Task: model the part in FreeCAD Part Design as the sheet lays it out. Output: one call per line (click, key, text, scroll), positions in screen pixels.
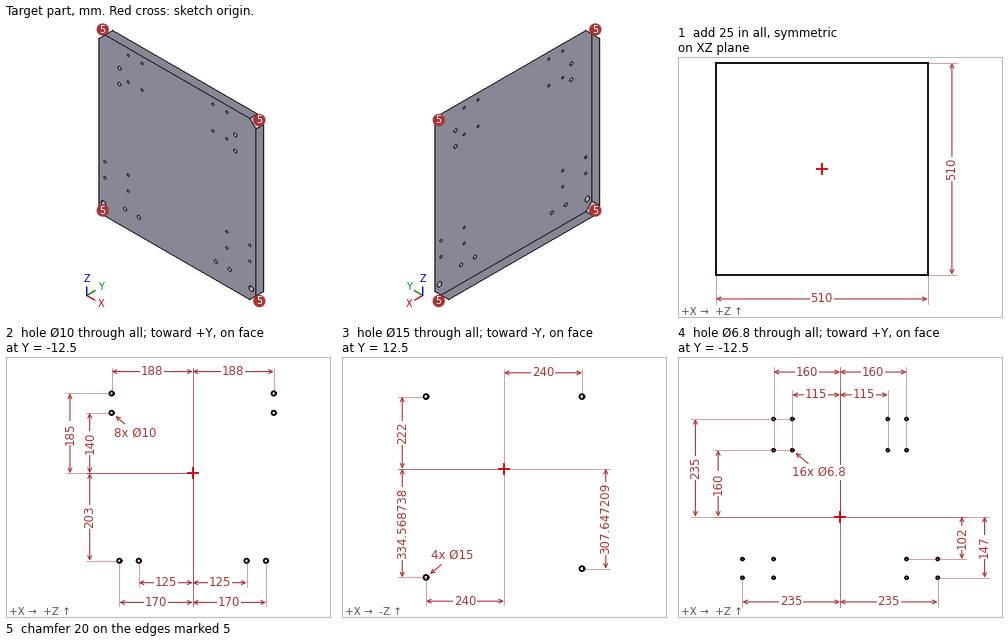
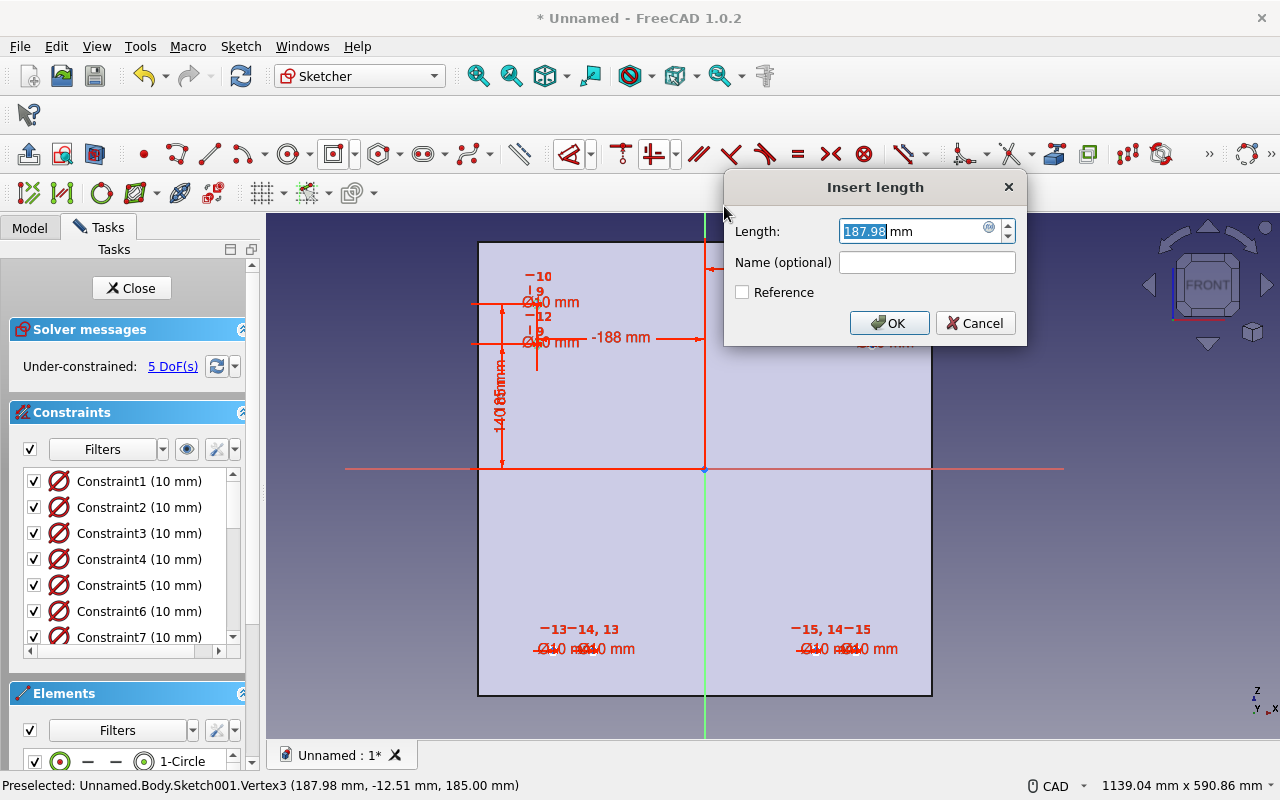
text(188)
key(Return)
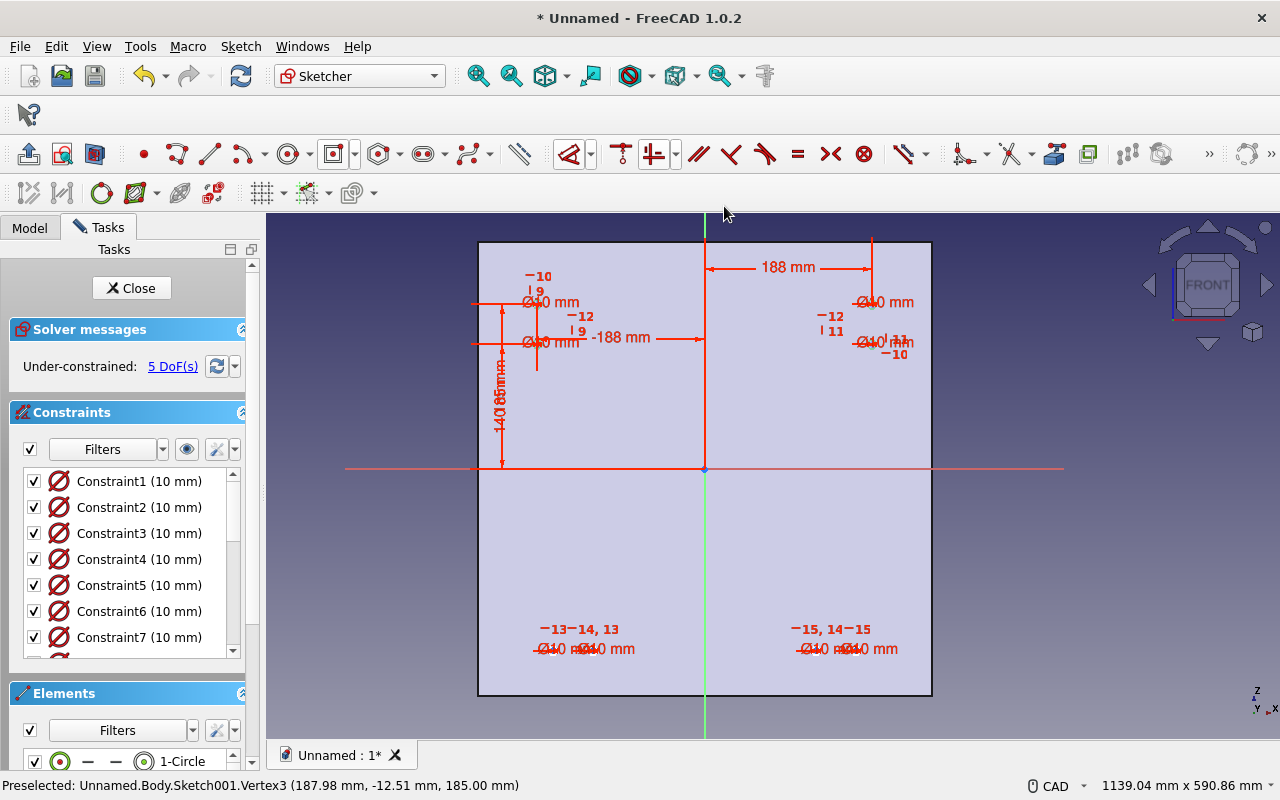
click(553, 651)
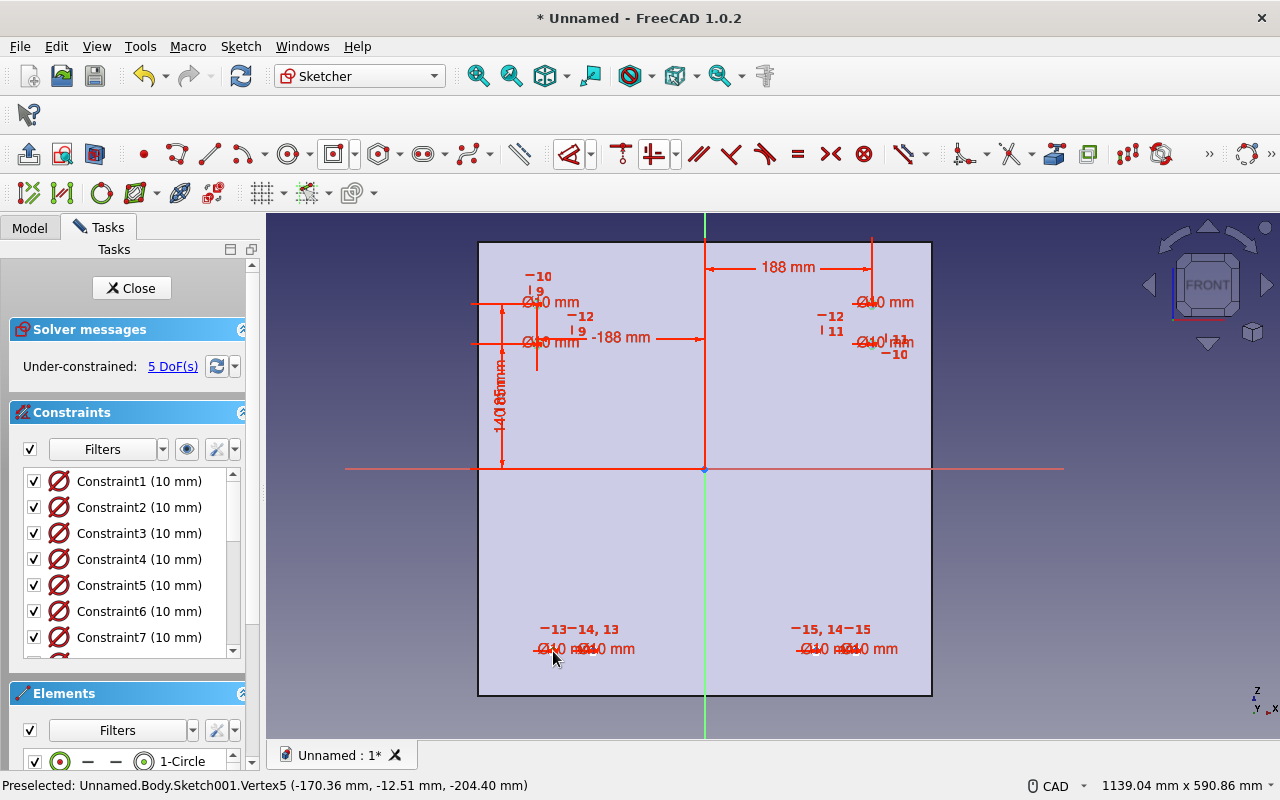
click(590, 154)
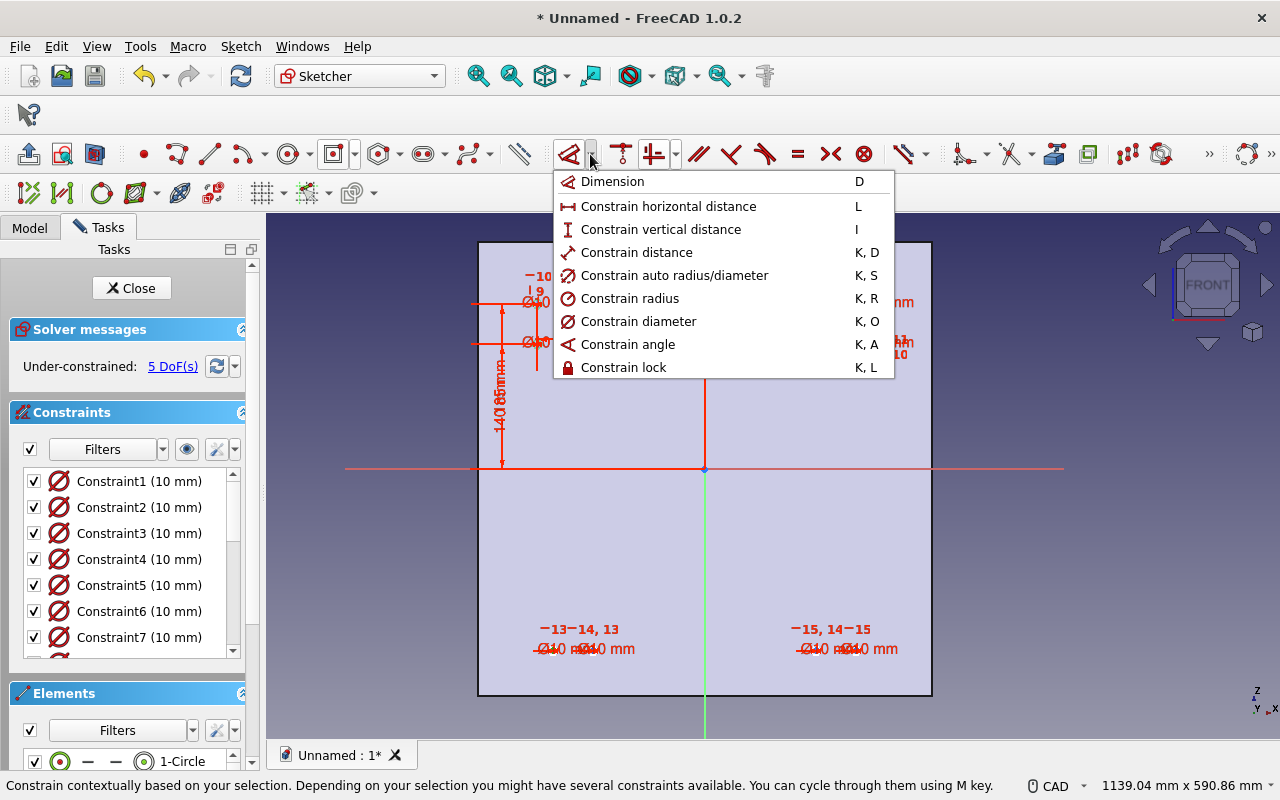
click(724, 206)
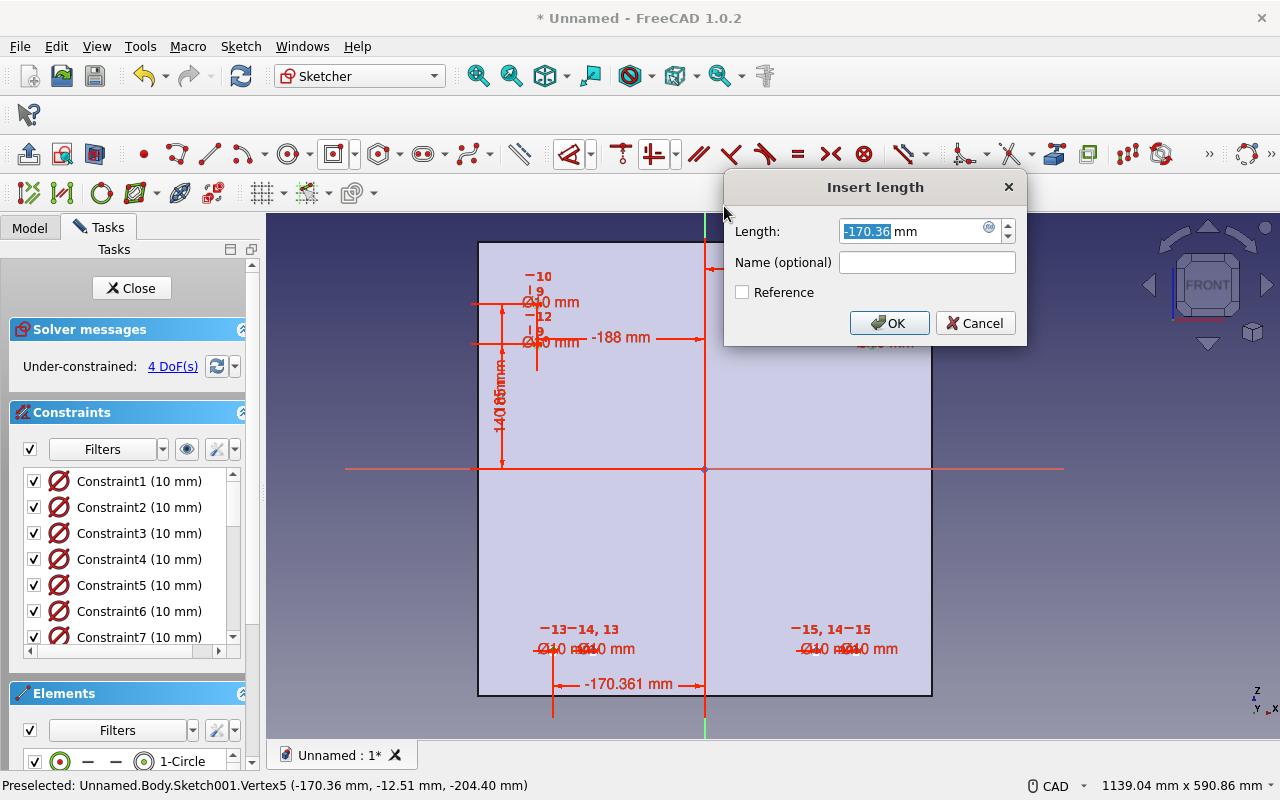
text(-170)
key(Return)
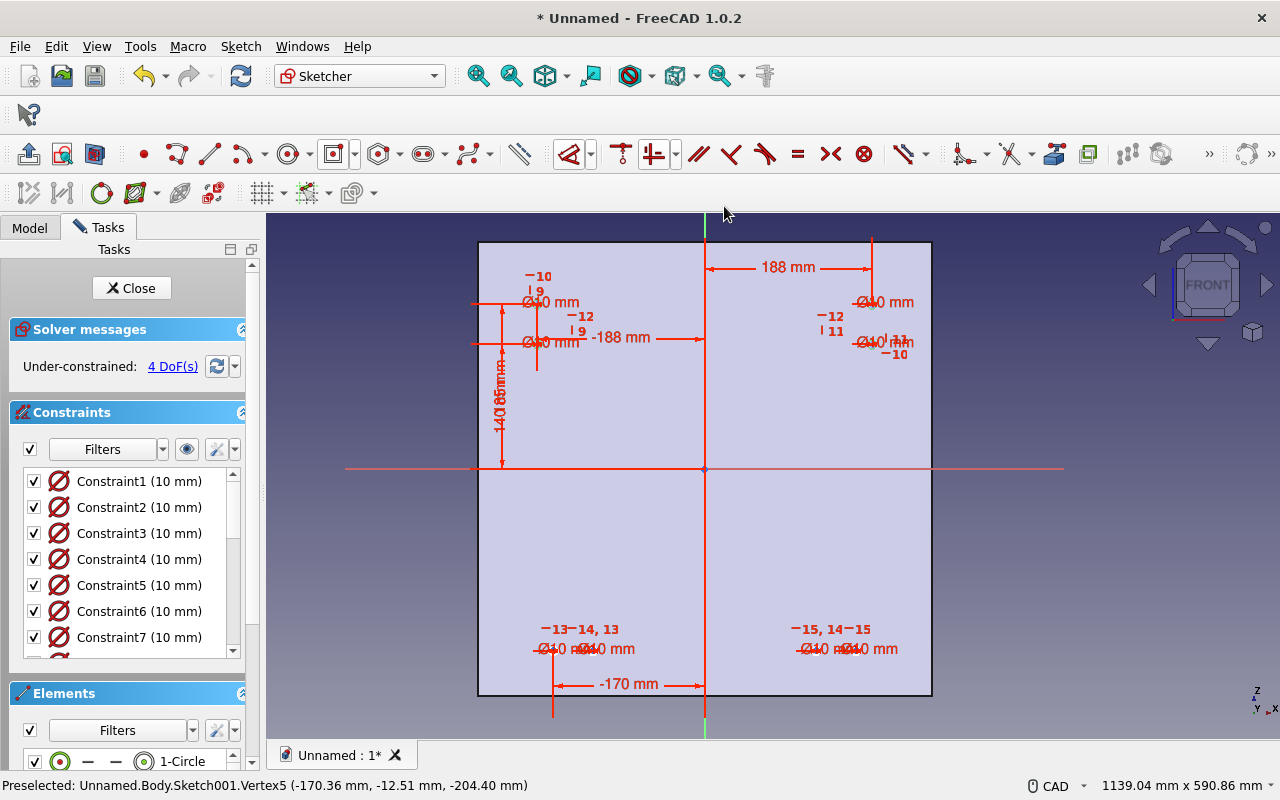
click(553, 651)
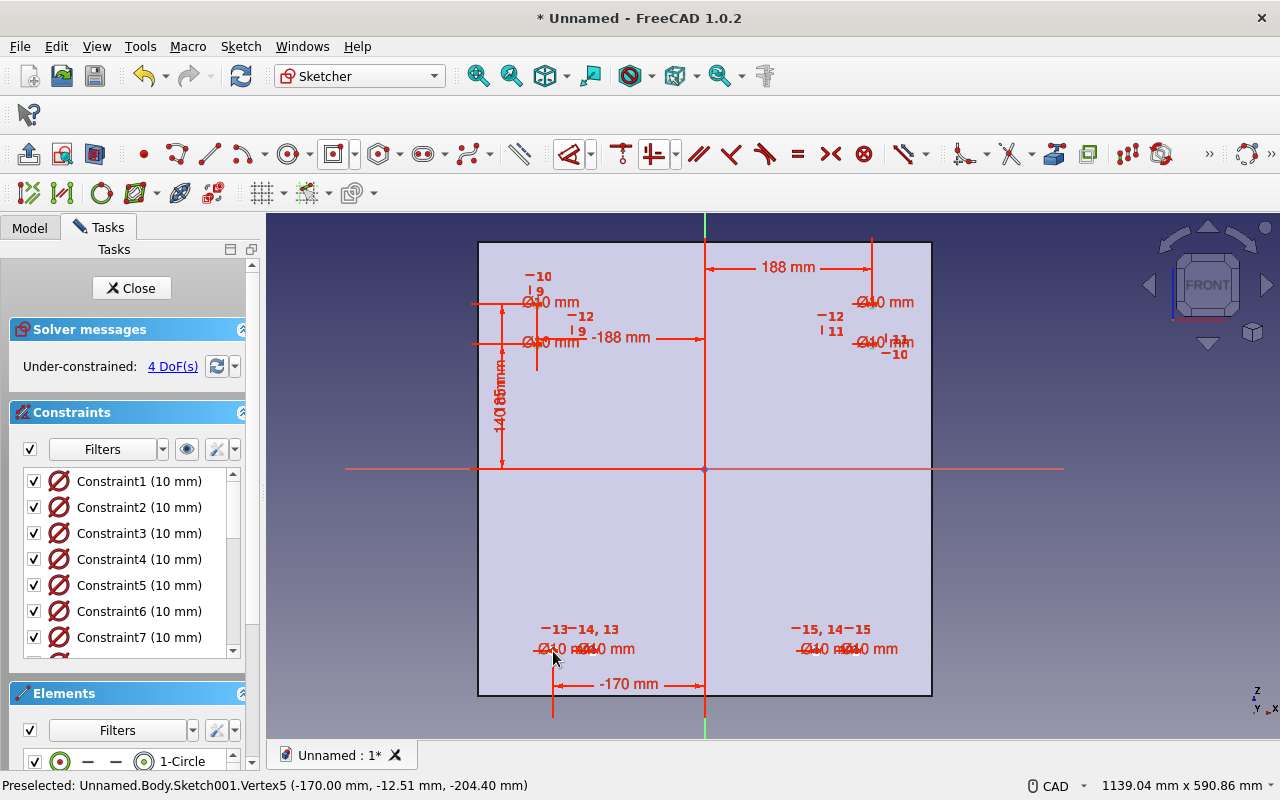
key(i)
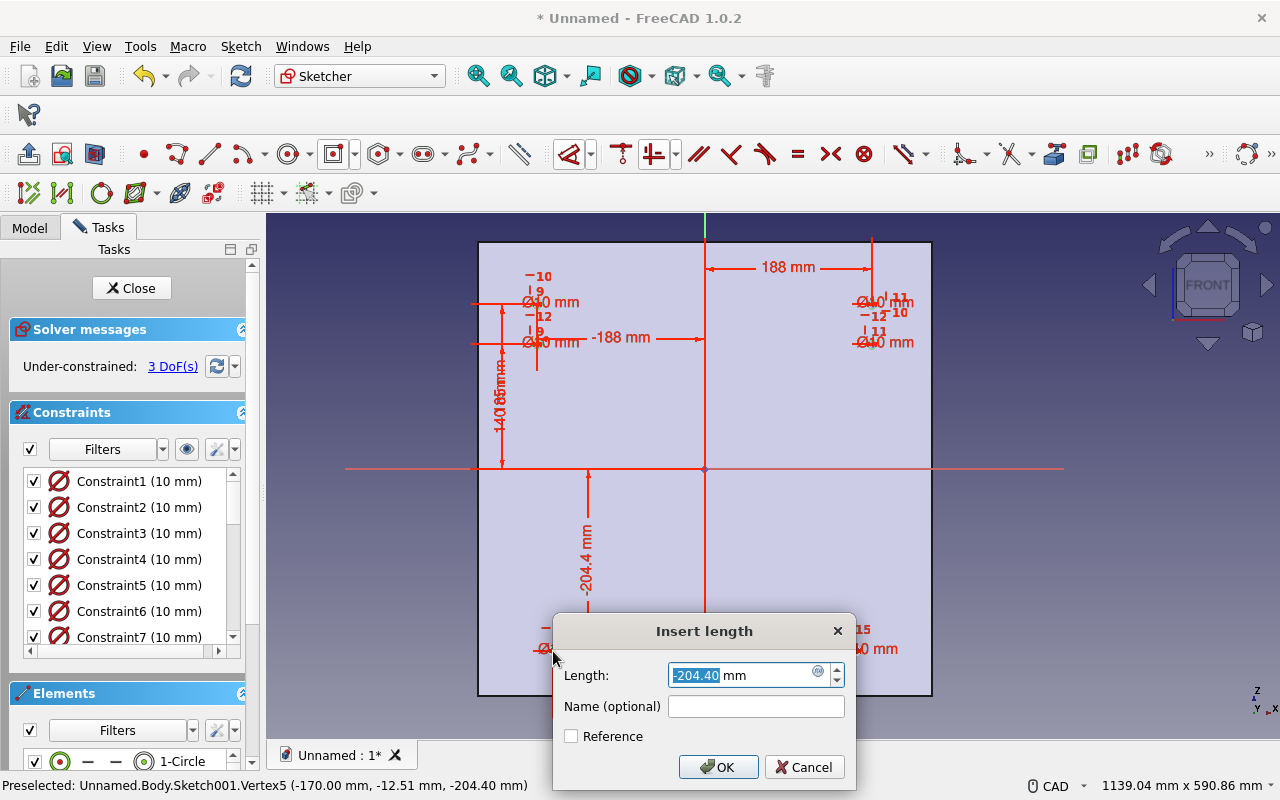
text(-203)
key(Return)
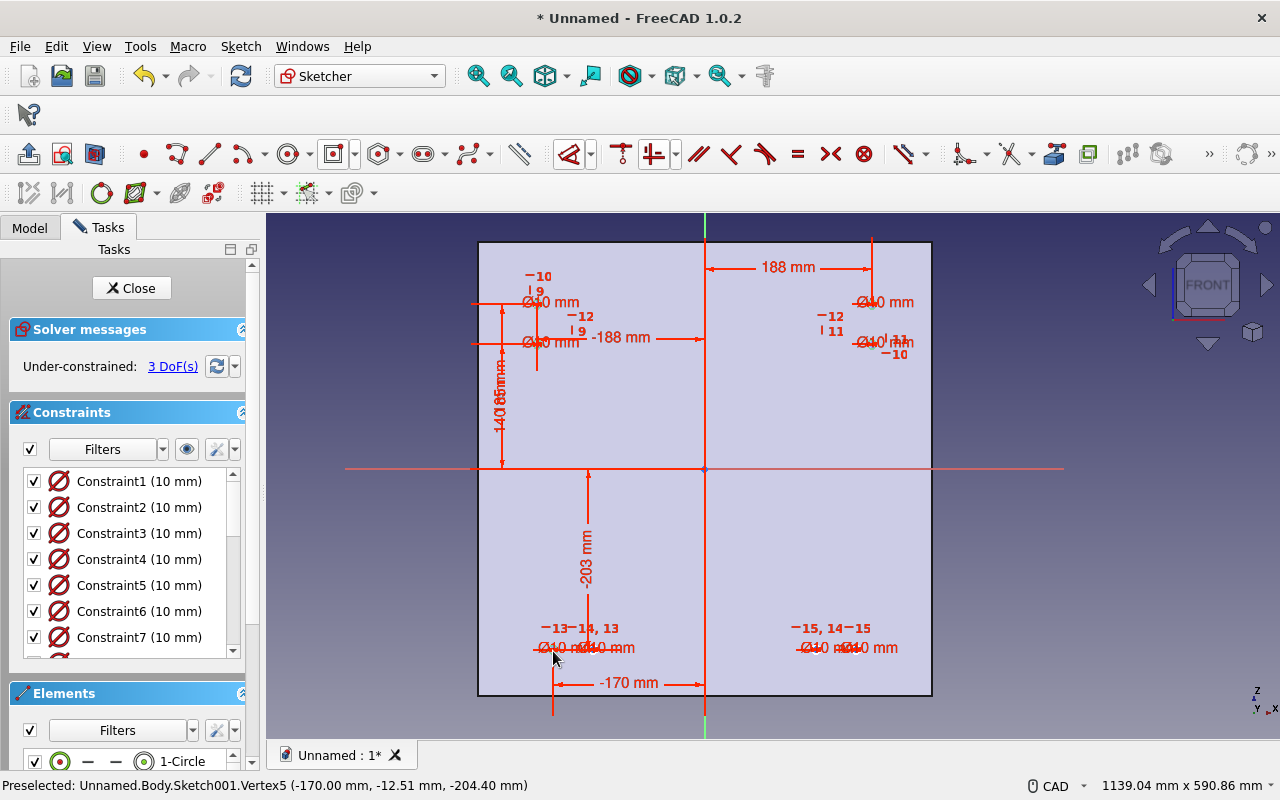
click(593, 650)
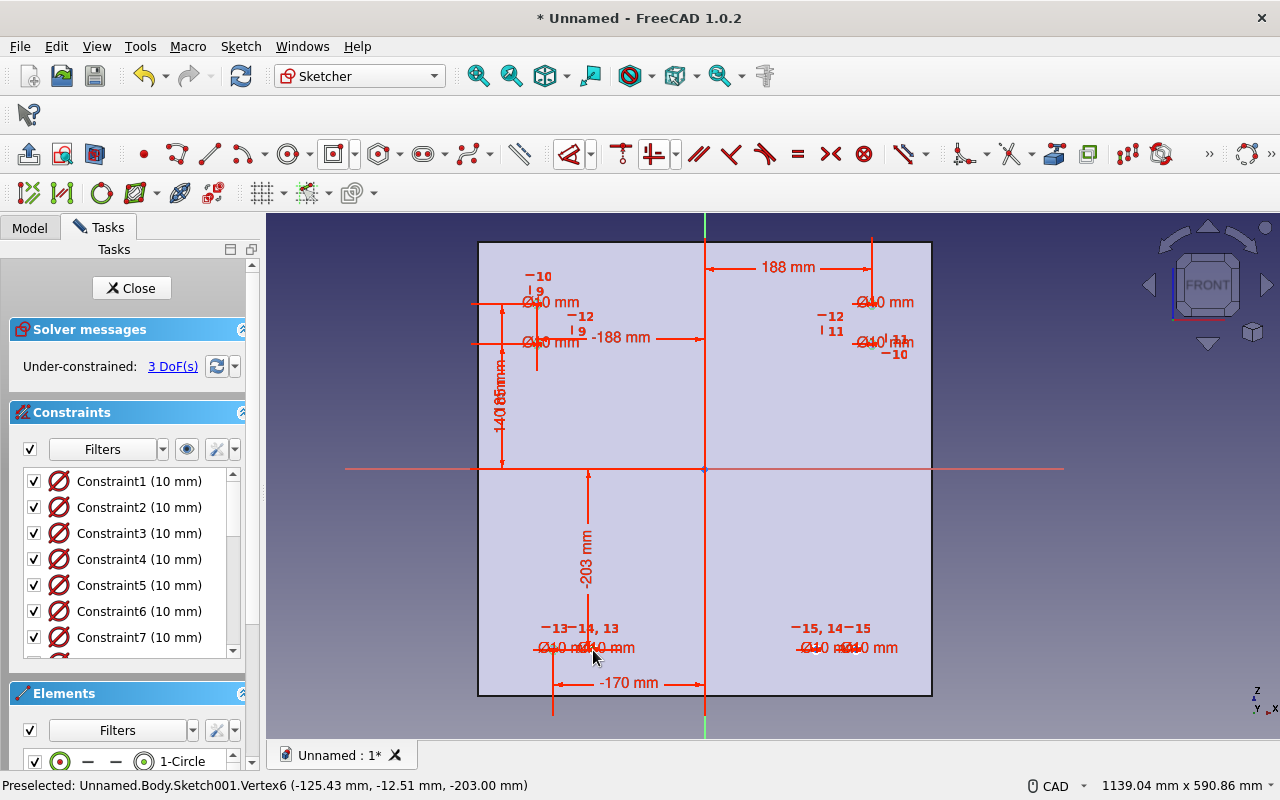
key(l)